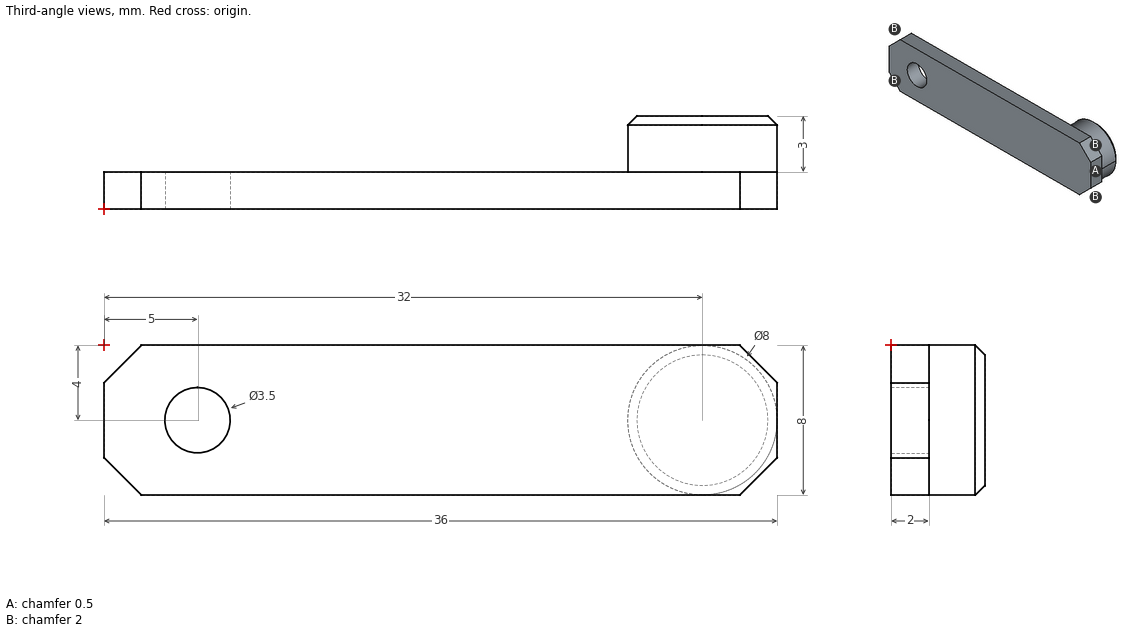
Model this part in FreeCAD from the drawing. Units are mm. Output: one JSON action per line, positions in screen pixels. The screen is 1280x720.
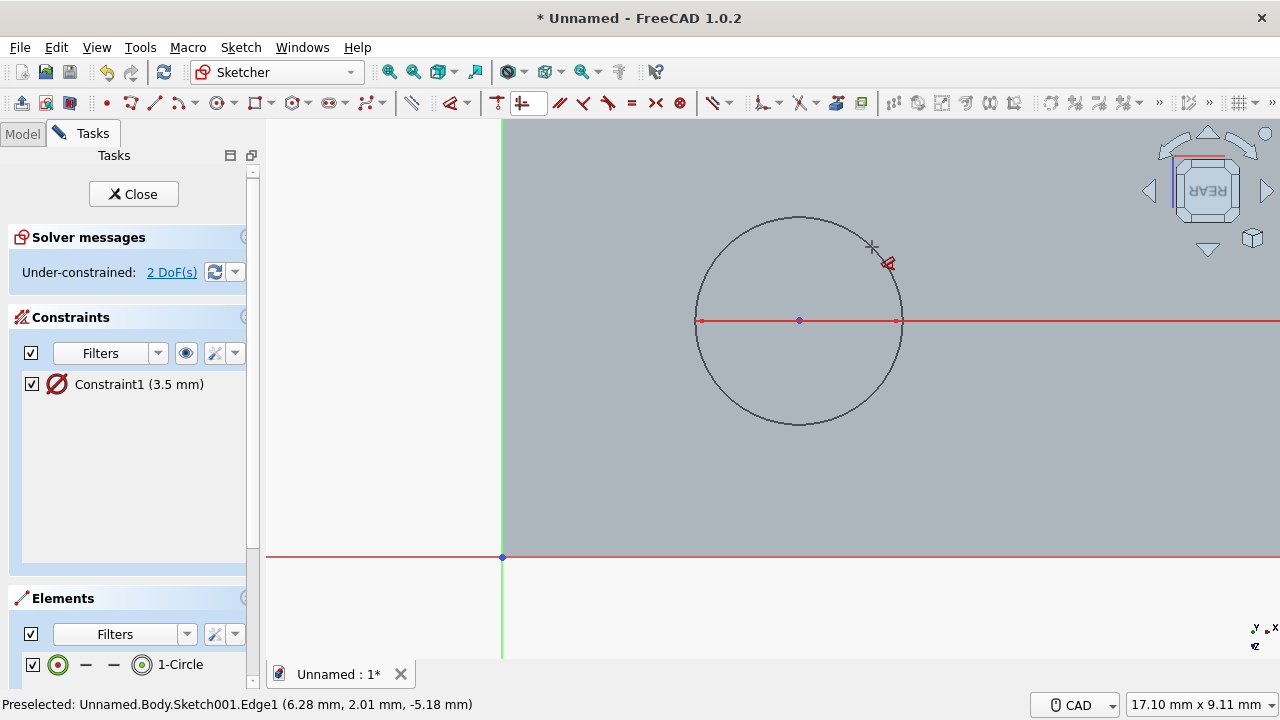
{"action": "left_click", "coordinate": [799, 321]}
{"action": "left_click", "coordinate": [651, 591]}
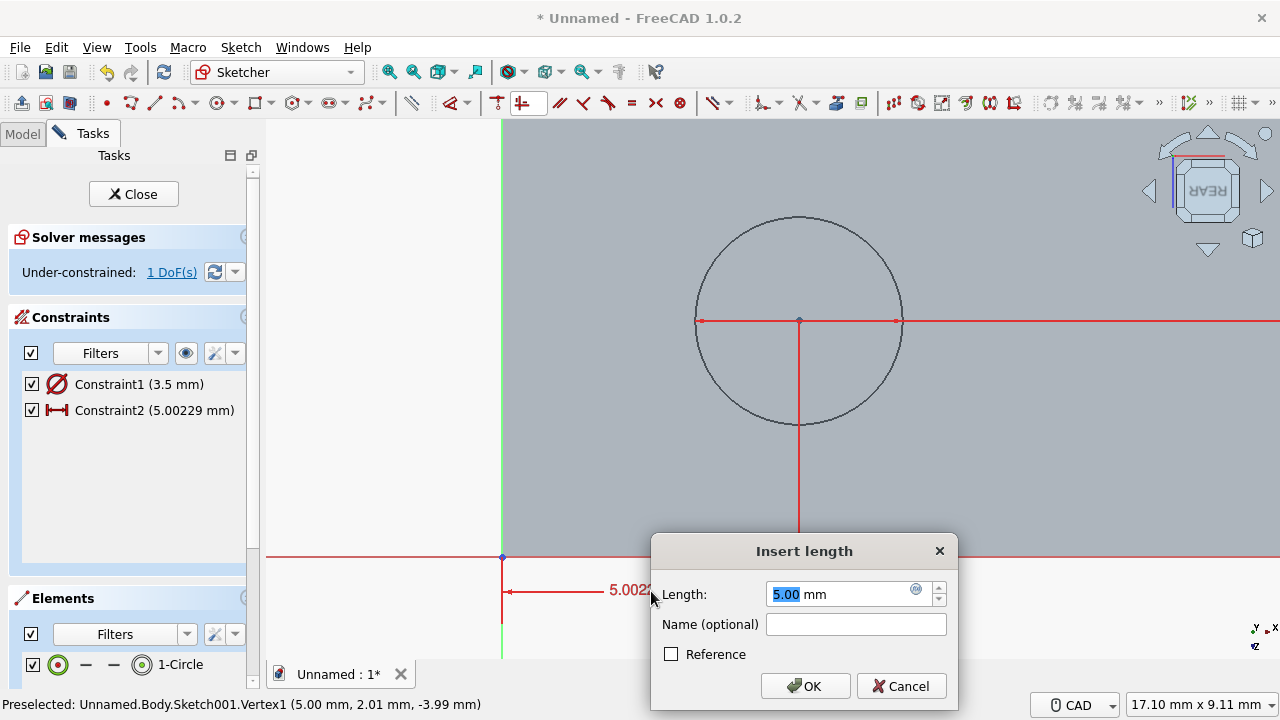
{"action": "type", "text": "5"}
{"action": "key", "text": "Return"}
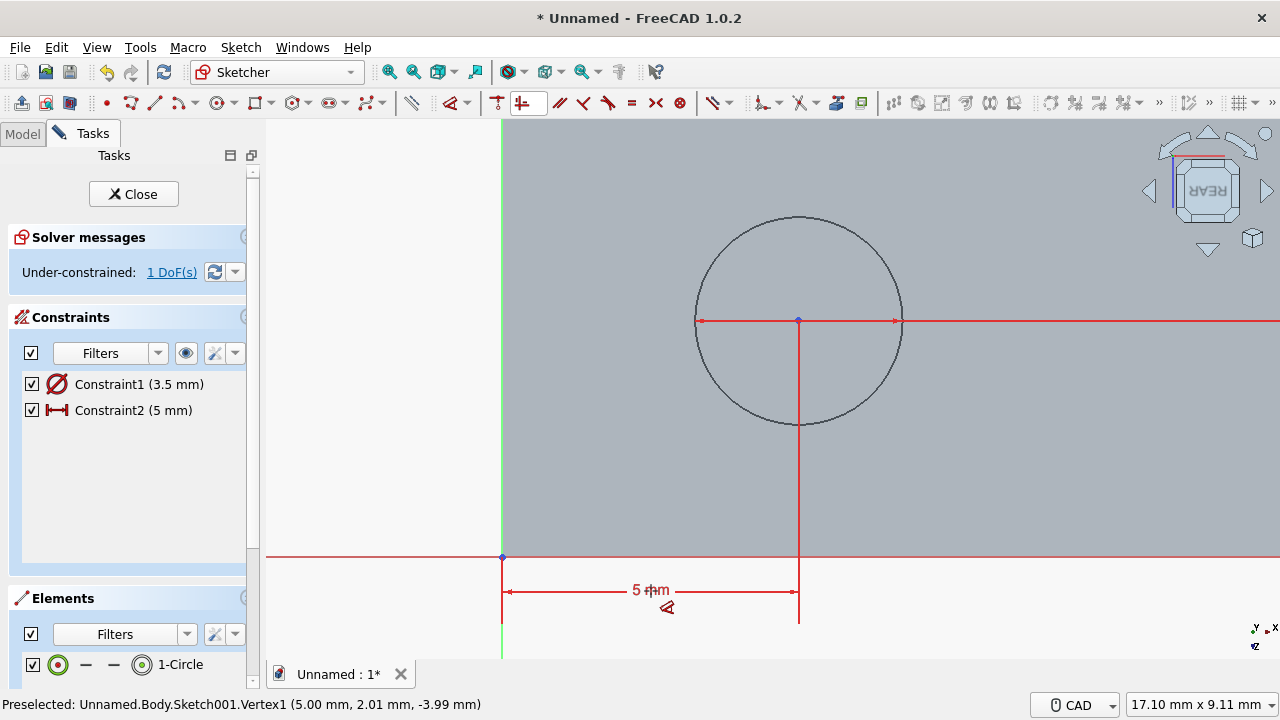
{"action": "left_click", "coordinate": [799, 321]}
{"action": "left_click", "coordinate": [468, 439]}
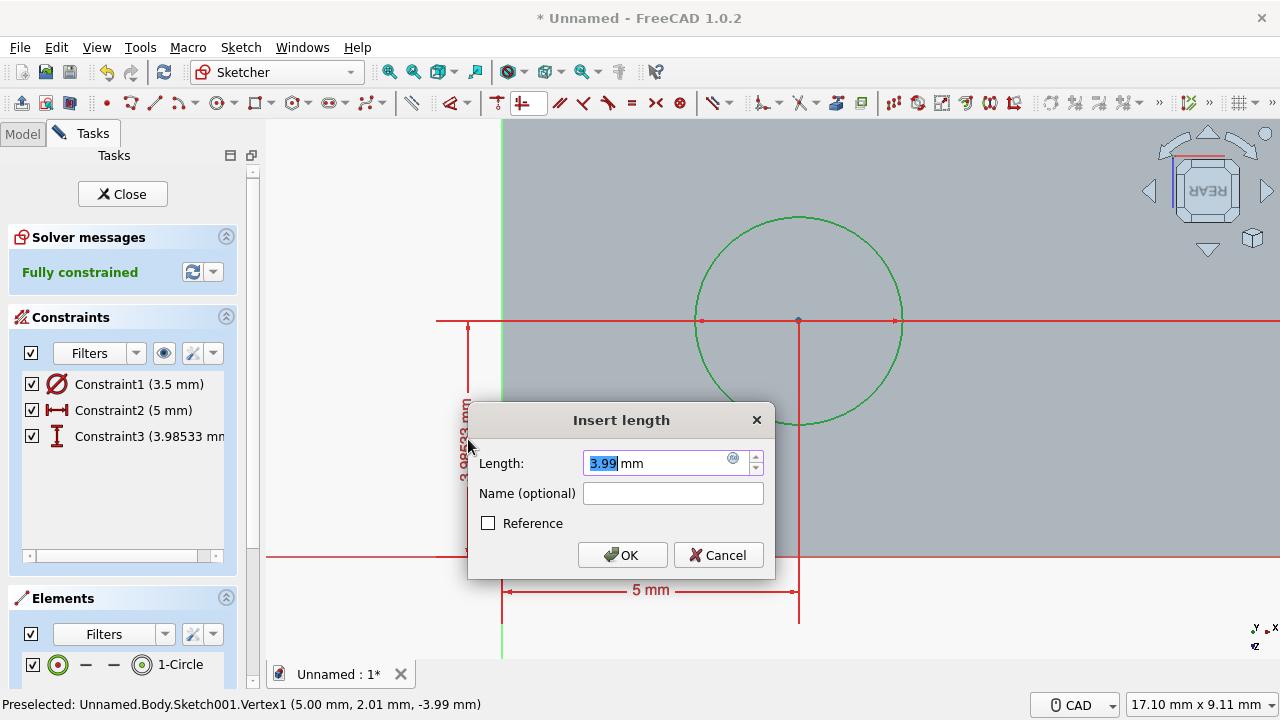
{"action": "type", "text": "4"}
{"action": "key", "text": "Return"}
{"action": "key", "text": "Escape"}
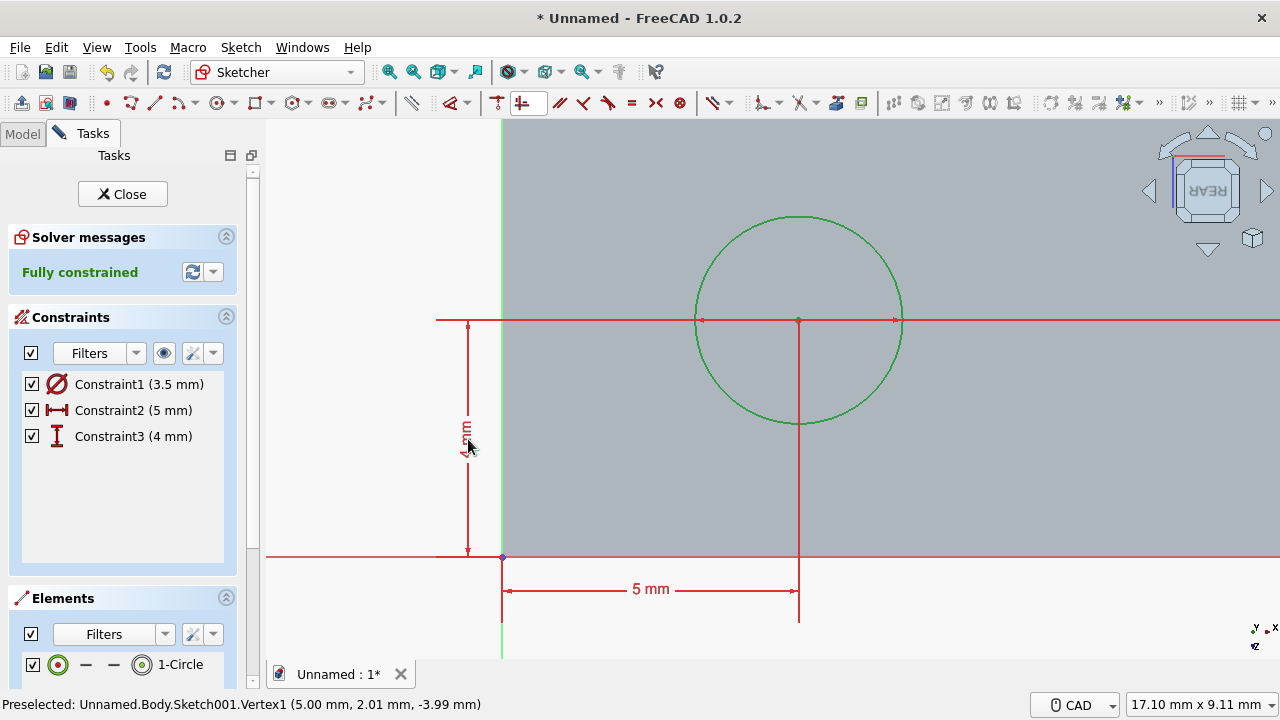
{"action": "left_click", "coordinate": [123, 194]}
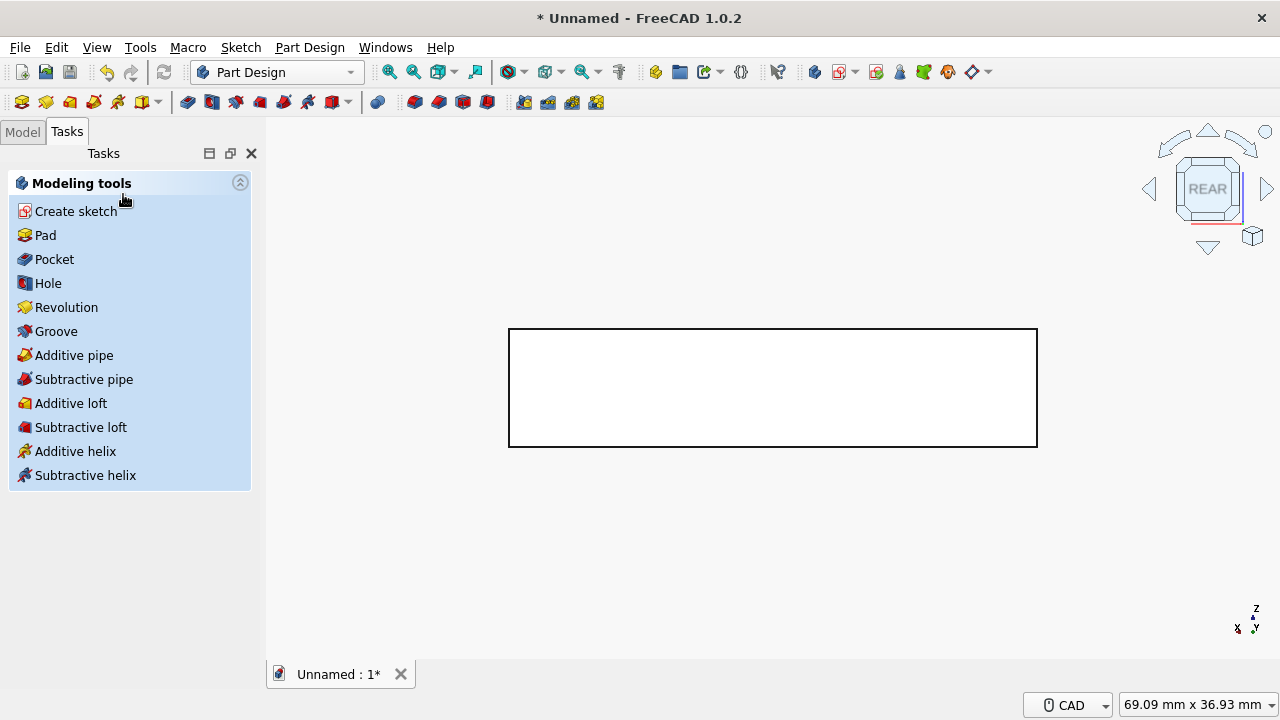
{"action": "left_click", "coordinate": [188, 102]}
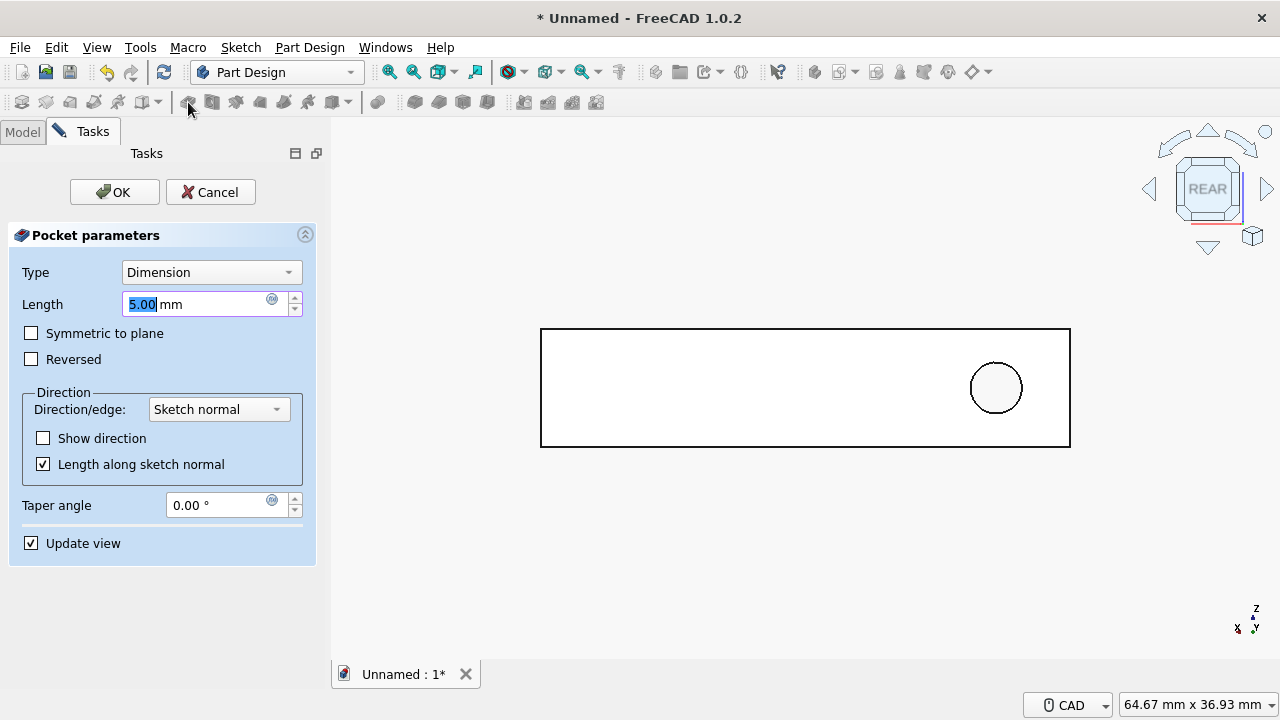
{"action": "left_click", "coordinate": [212, 272]}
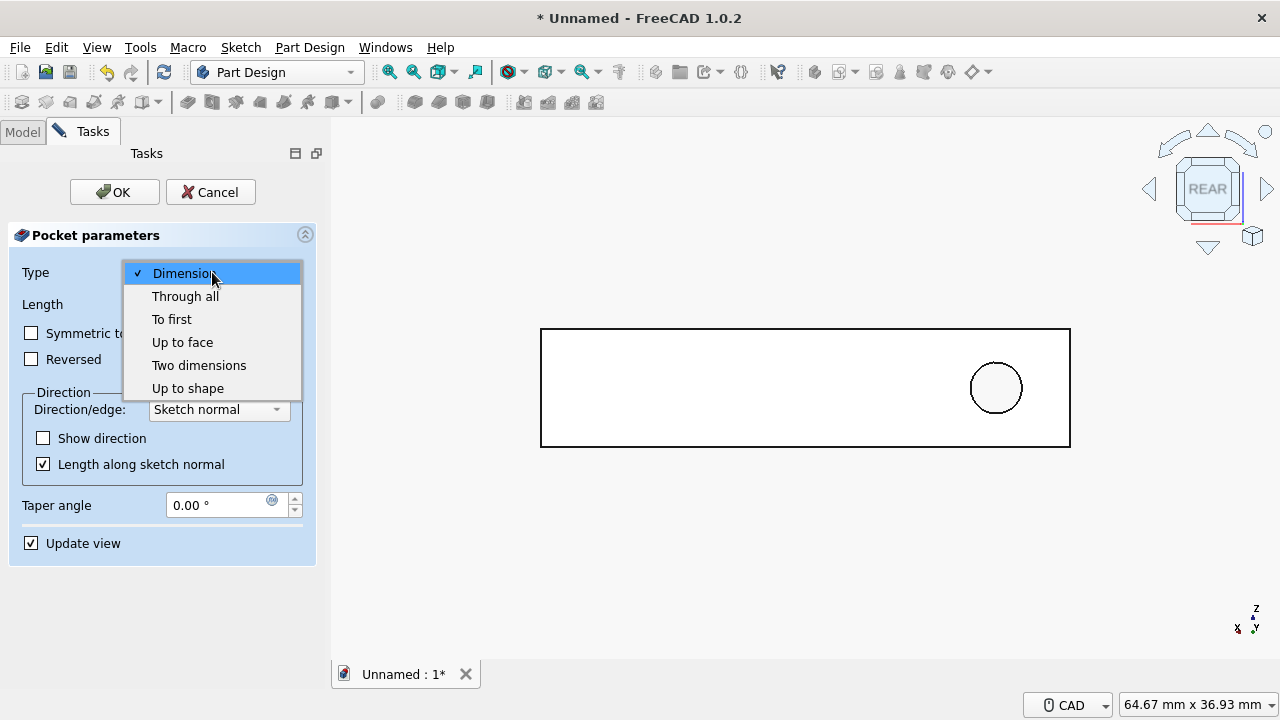
{"action": "left_click", "coordinate": [212, 296]}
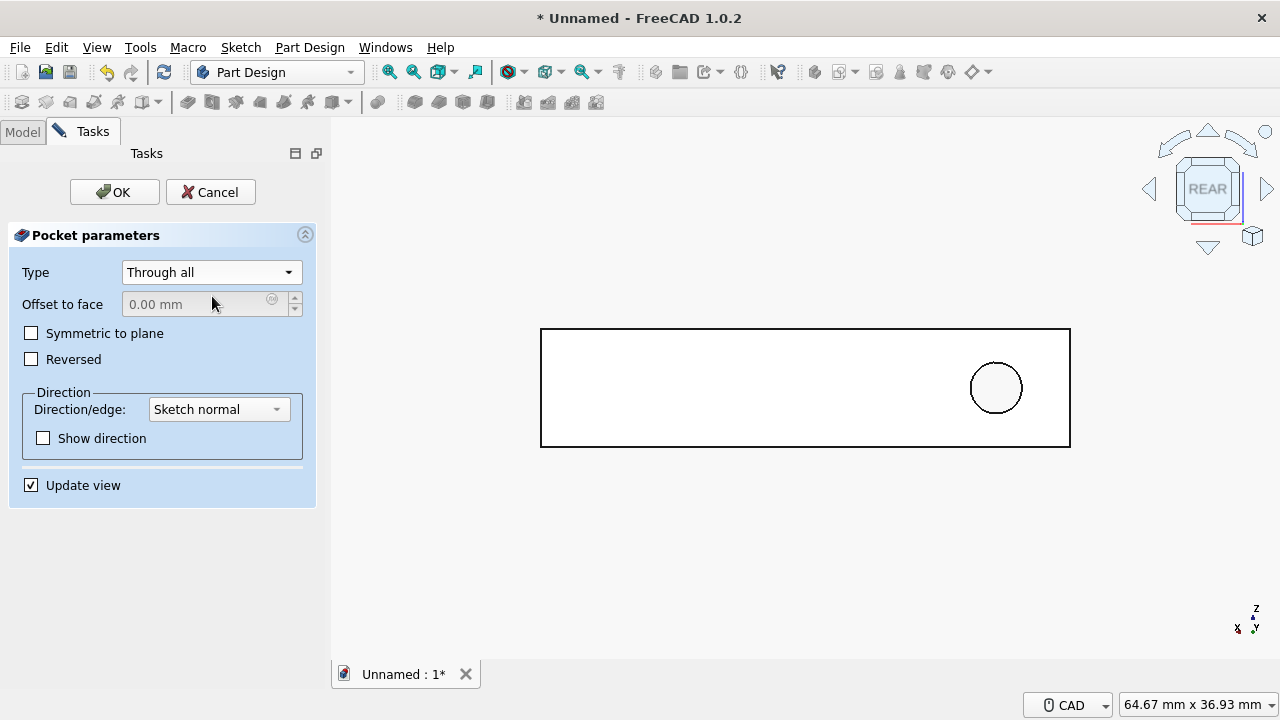
{"action": "left_click", "coordinate": [115, 192]}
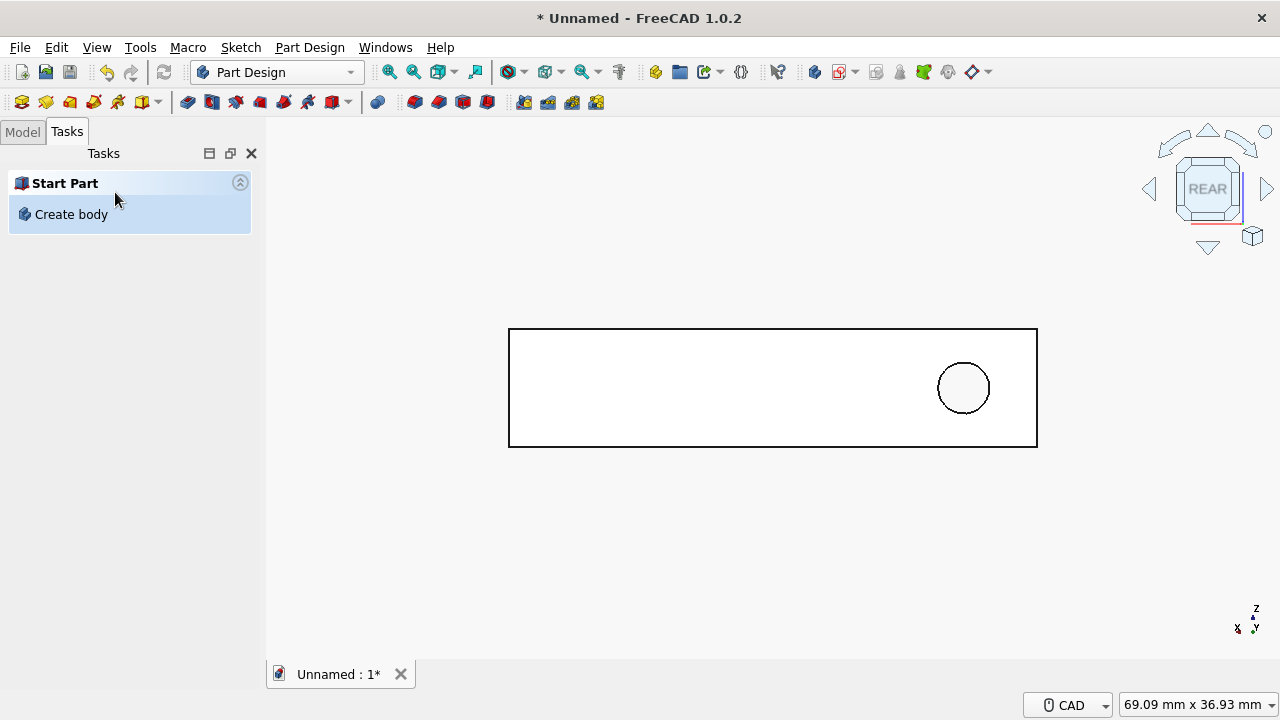
{"action": "left_click", "coordinate": [622, 387]}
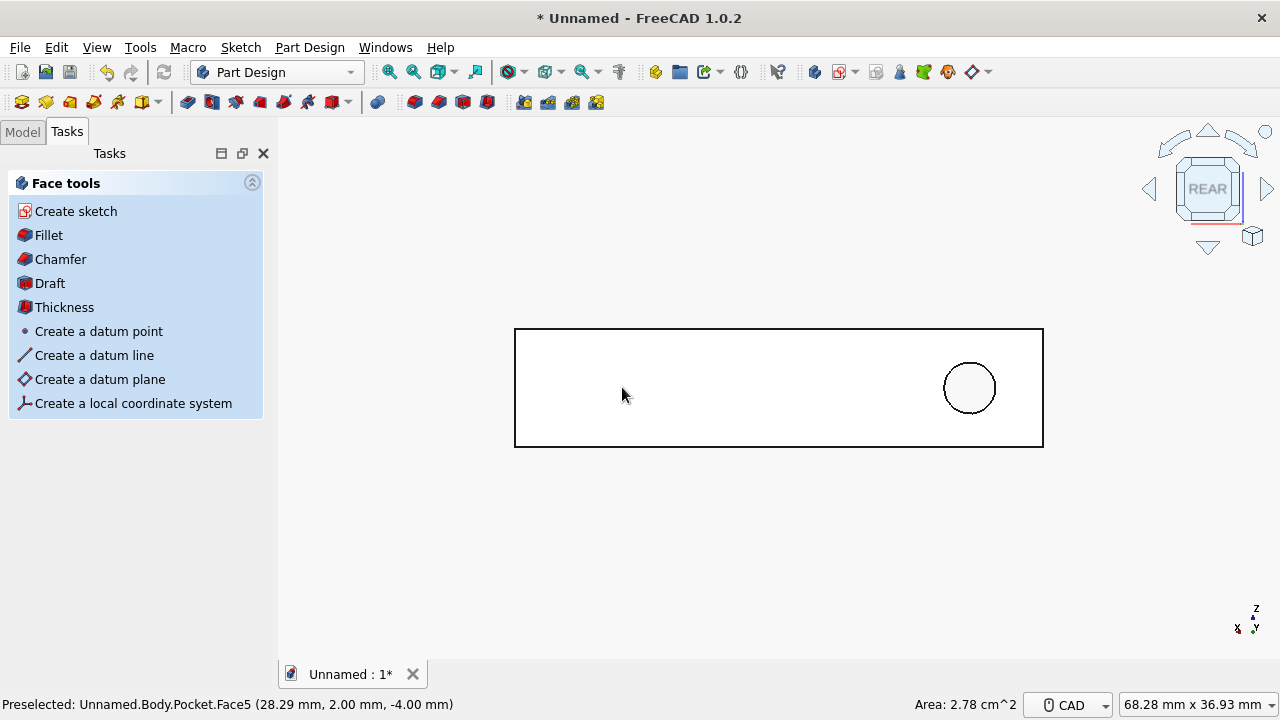
{"action": "left_click", "coordinate": [840, 72]}